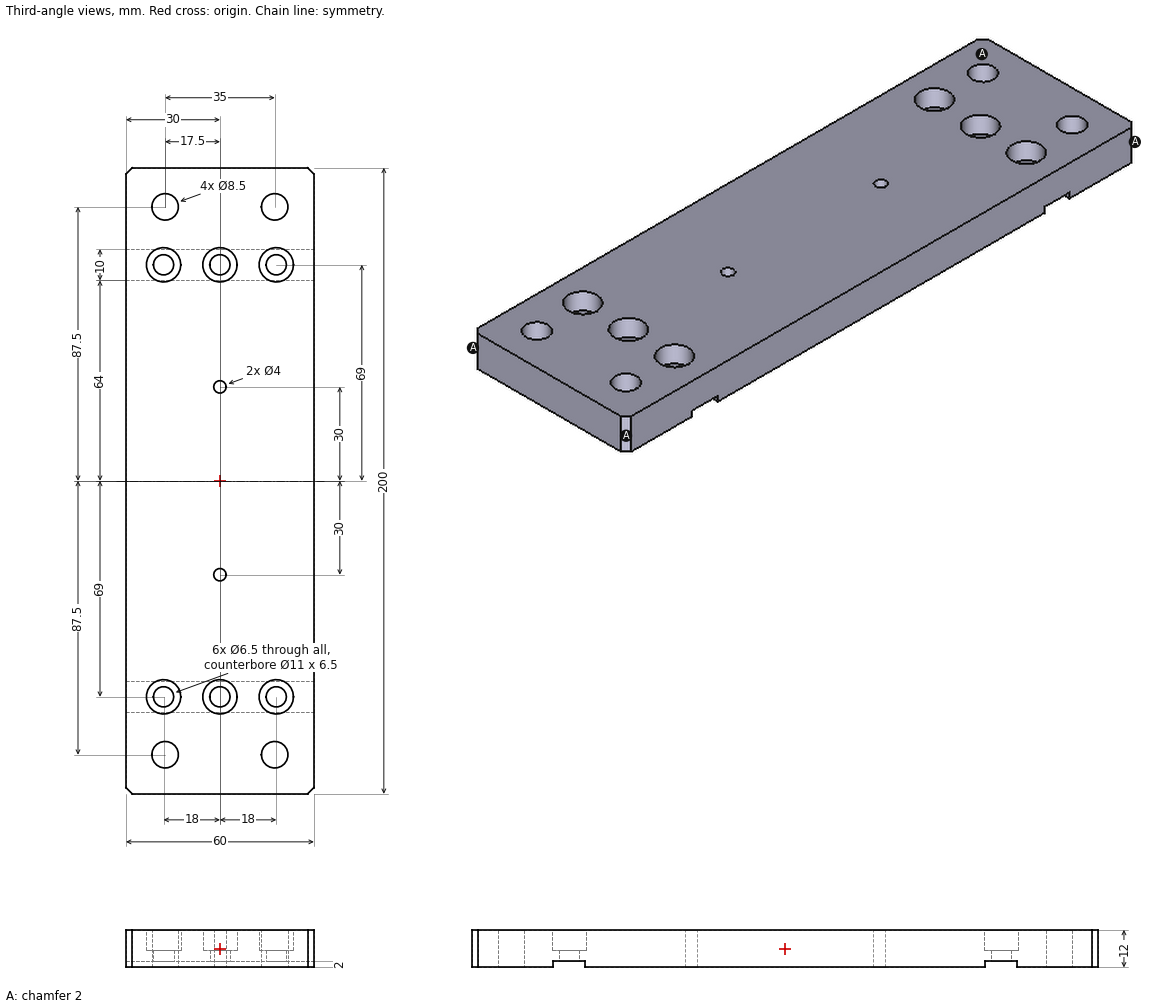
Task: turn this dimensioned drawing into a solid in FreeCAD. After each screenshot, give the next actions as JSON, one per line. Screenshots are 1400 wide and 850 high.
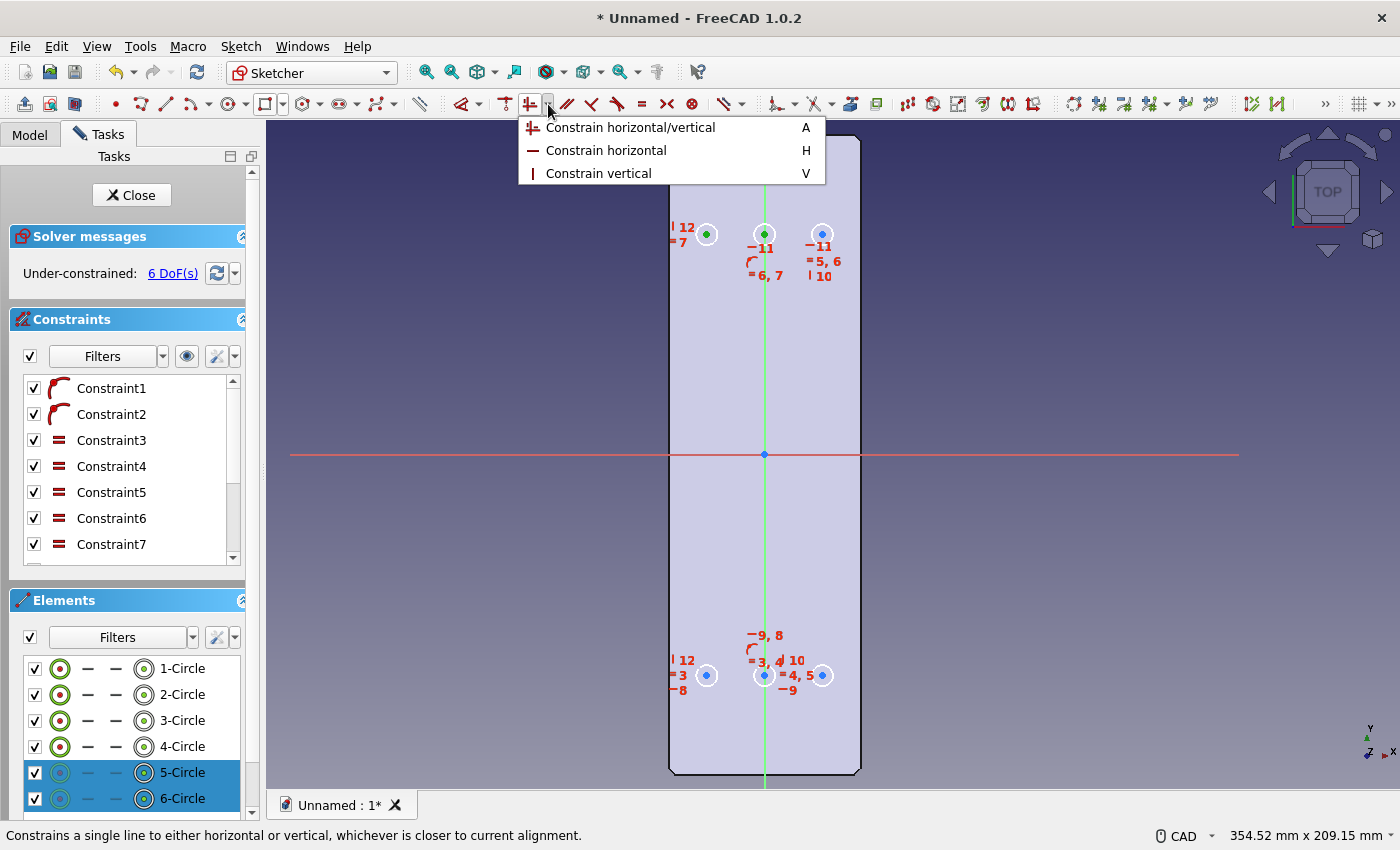
{"action": "left_click", "coordinate": [672, 150]}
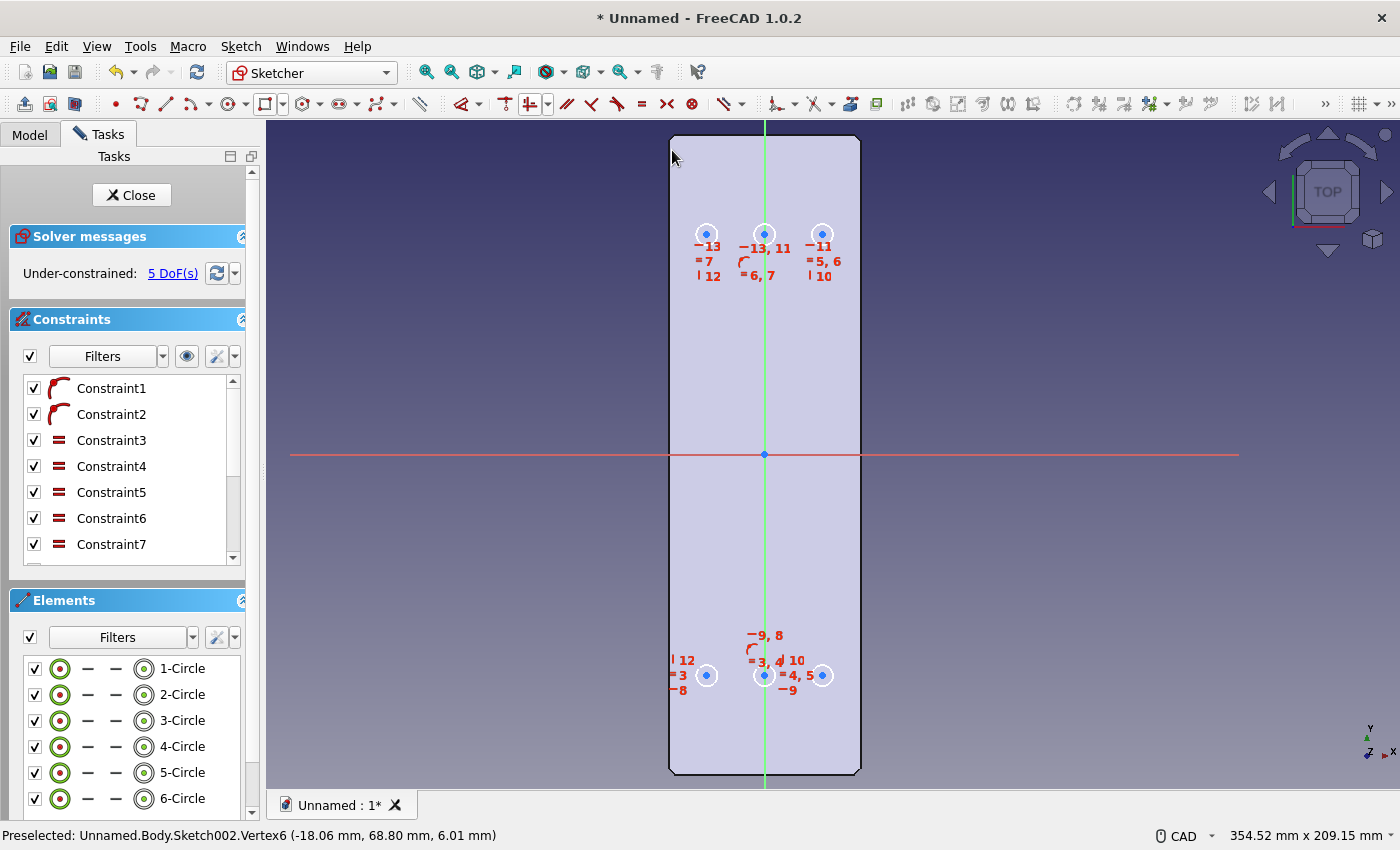
{"action": "left_click", "coordinate": [460, 104]}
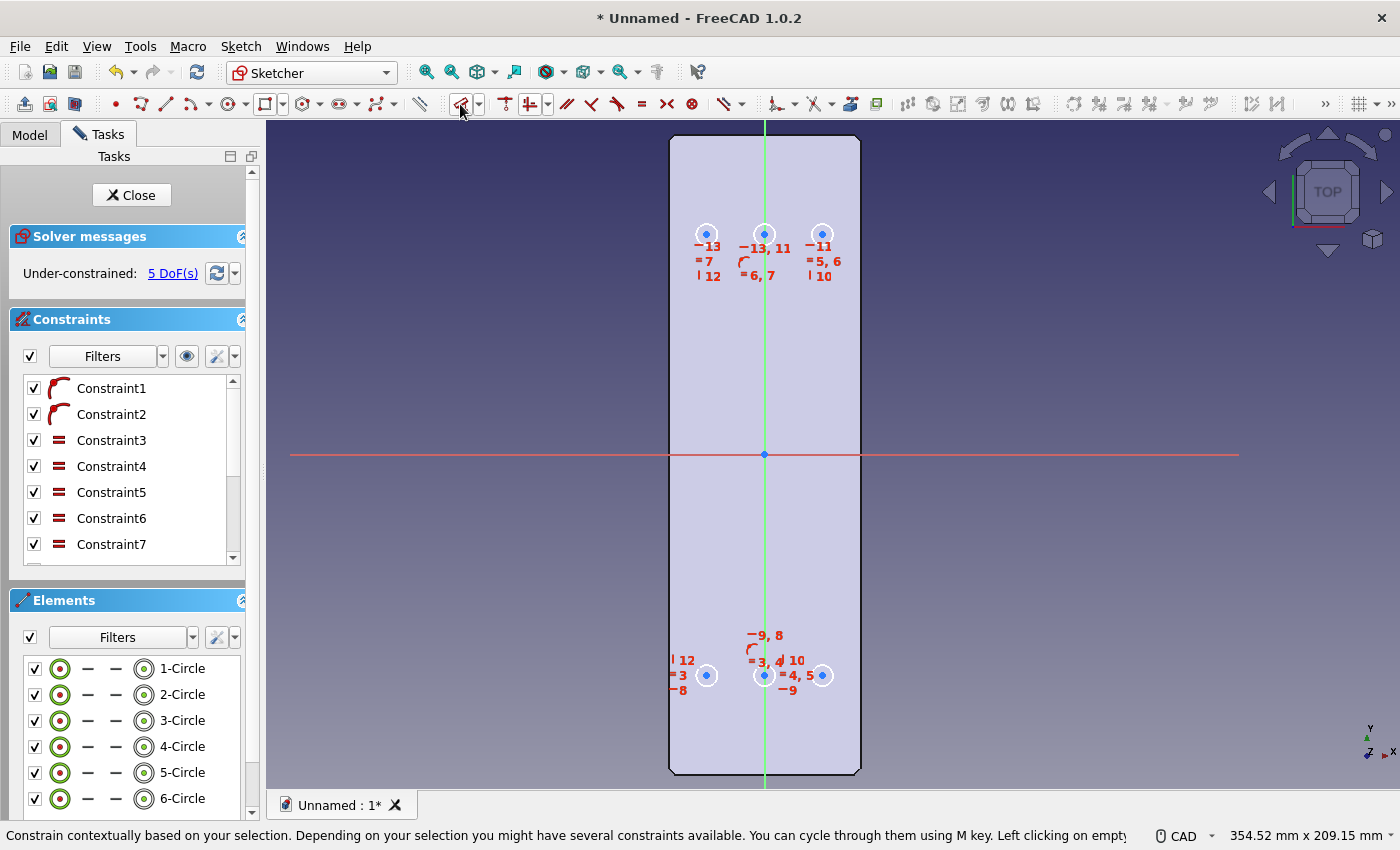
{"action": "scroll", "coordinate": [714, 668], "scroll_direction": "up", "scroll_amount": 4}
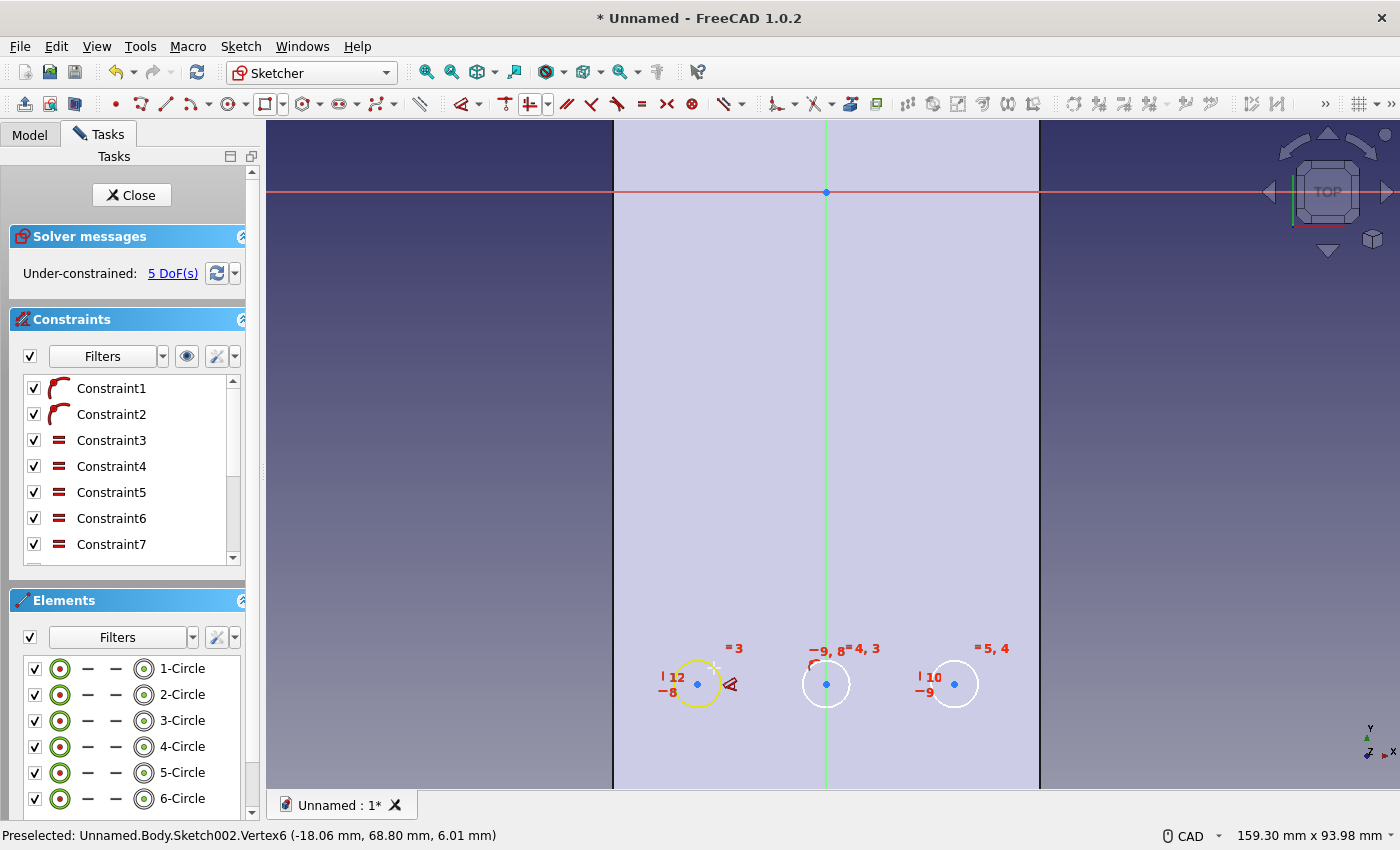
{"action": "left_click", "coordinate": [714, 668]}
{"action": "left_click", "coordinate": [737, 646]}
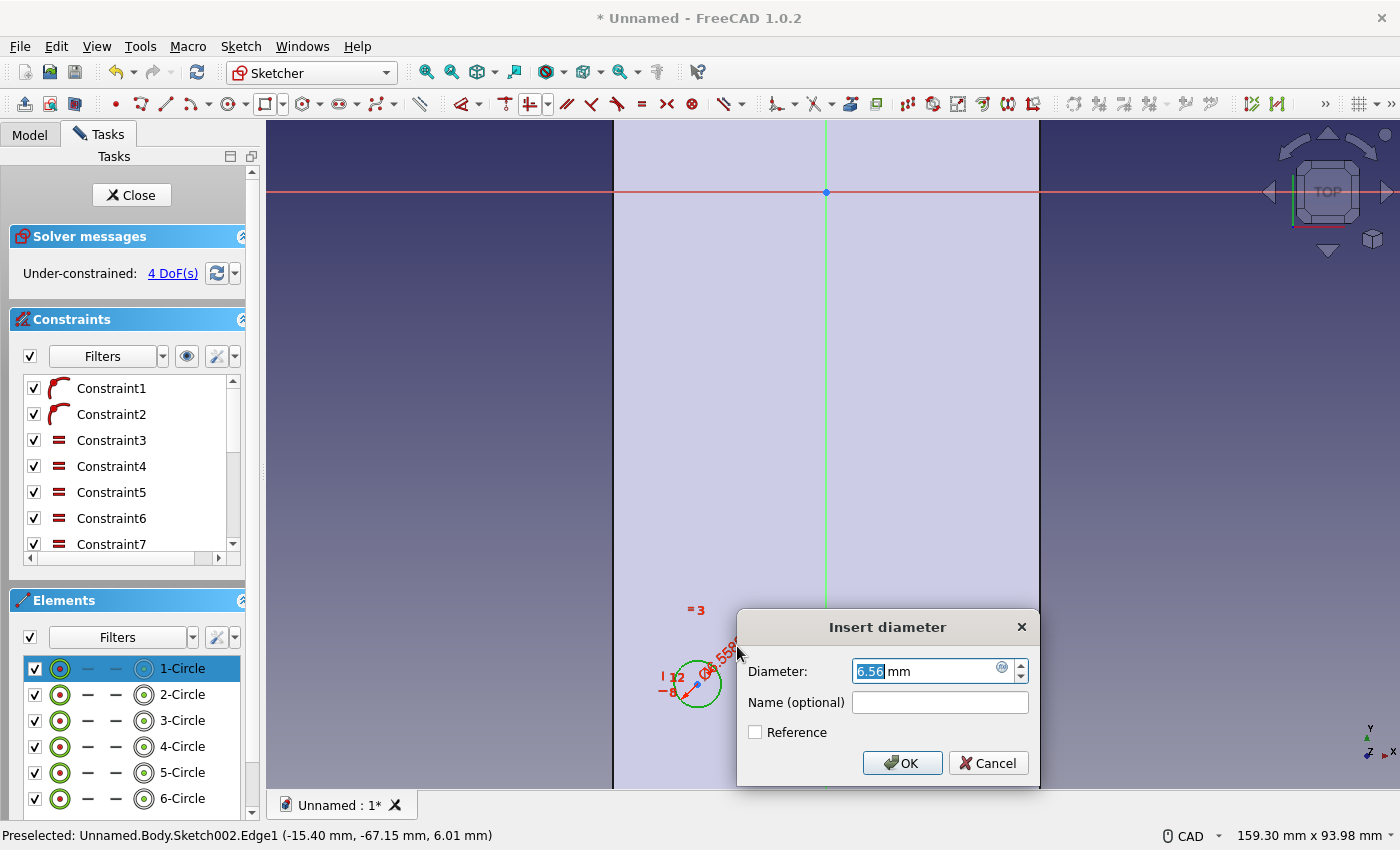
{"action": "type", "text": "6.5"}
{"action": "key", "text": "Return"}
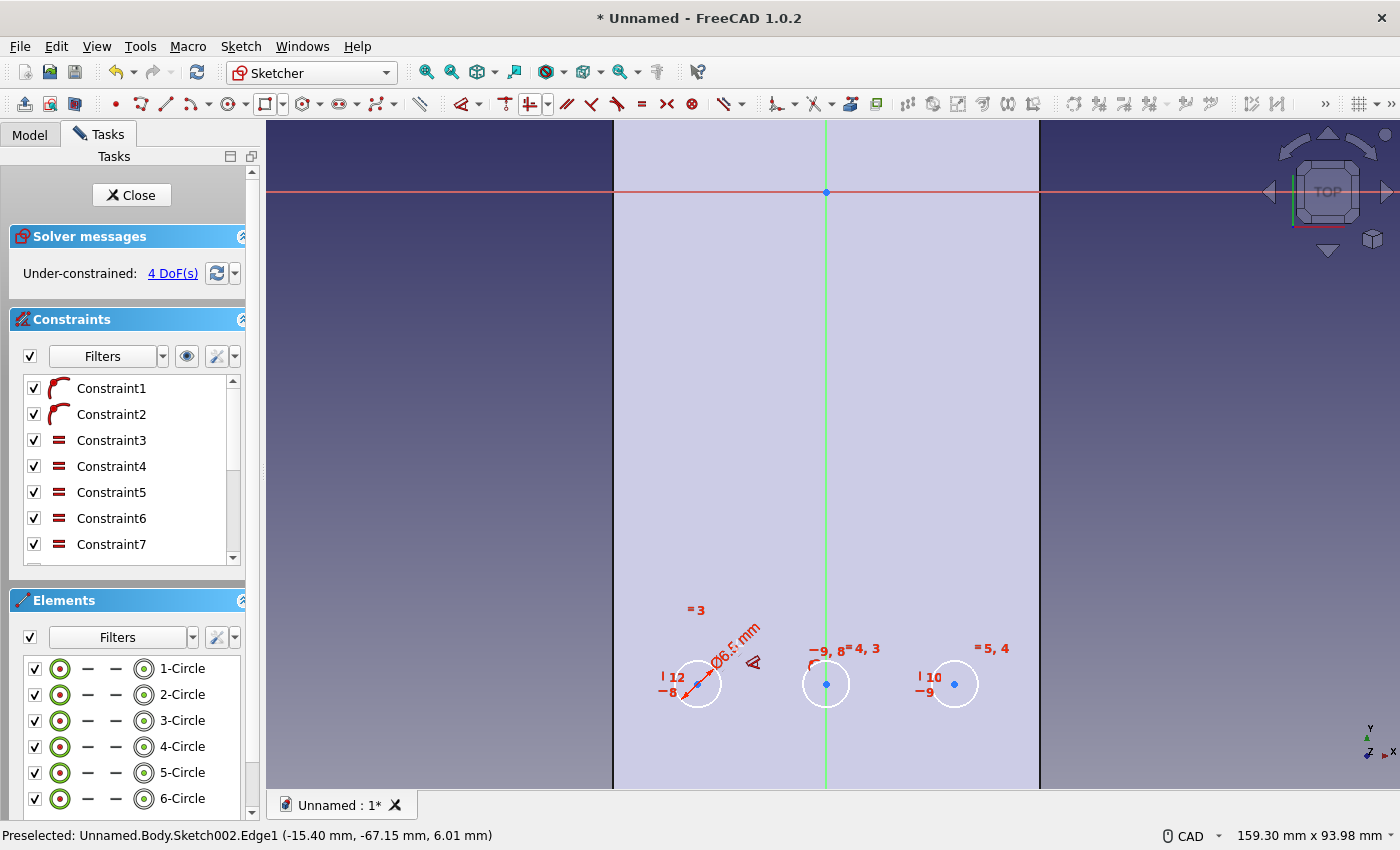
{"action": "left_click", "coordinate": [698, 684]}
{"action": "left_click", "coordinate": [762, 718]}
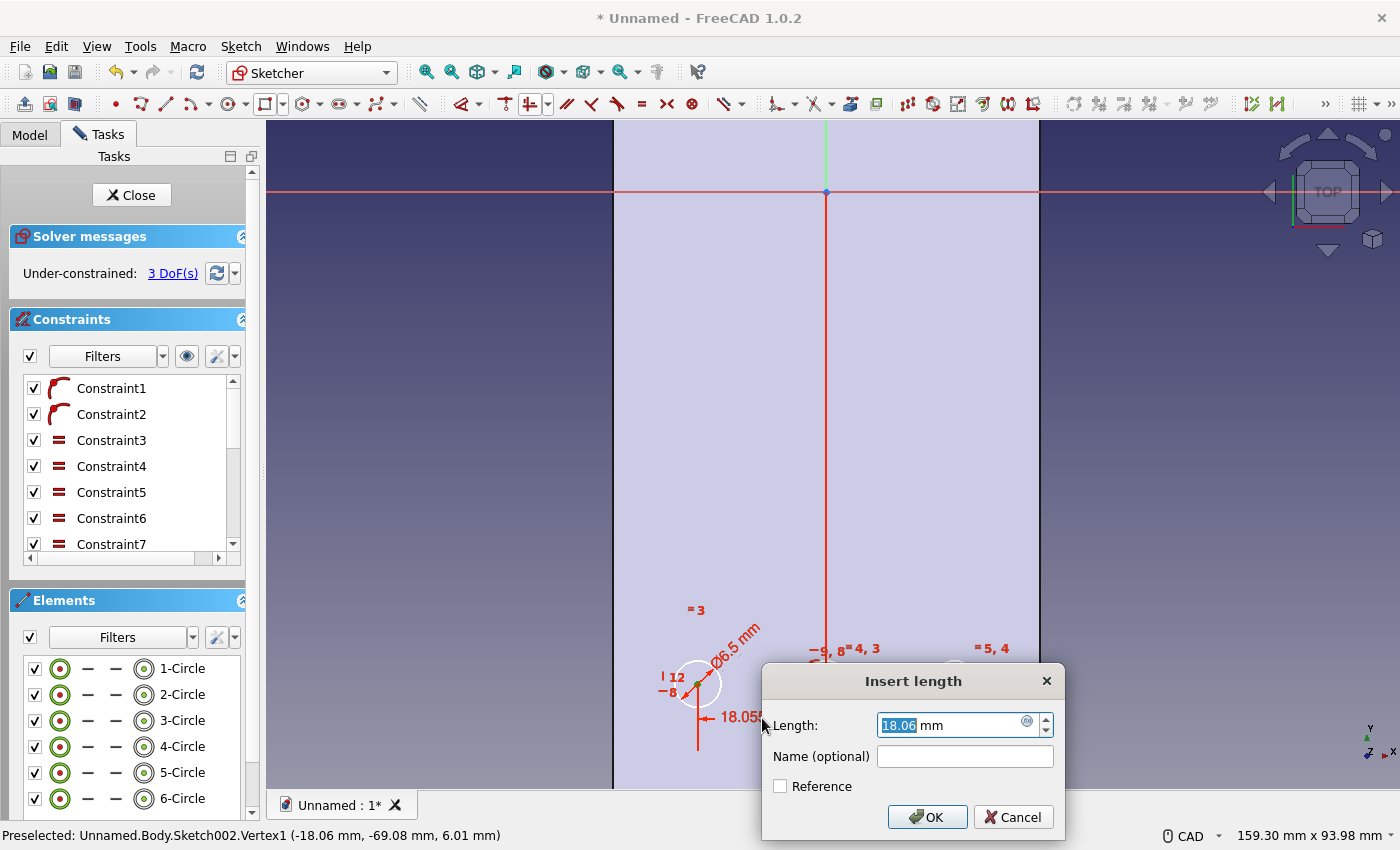
{"action": "type", "text": "18"}
{"action": "key", "text": "Return"}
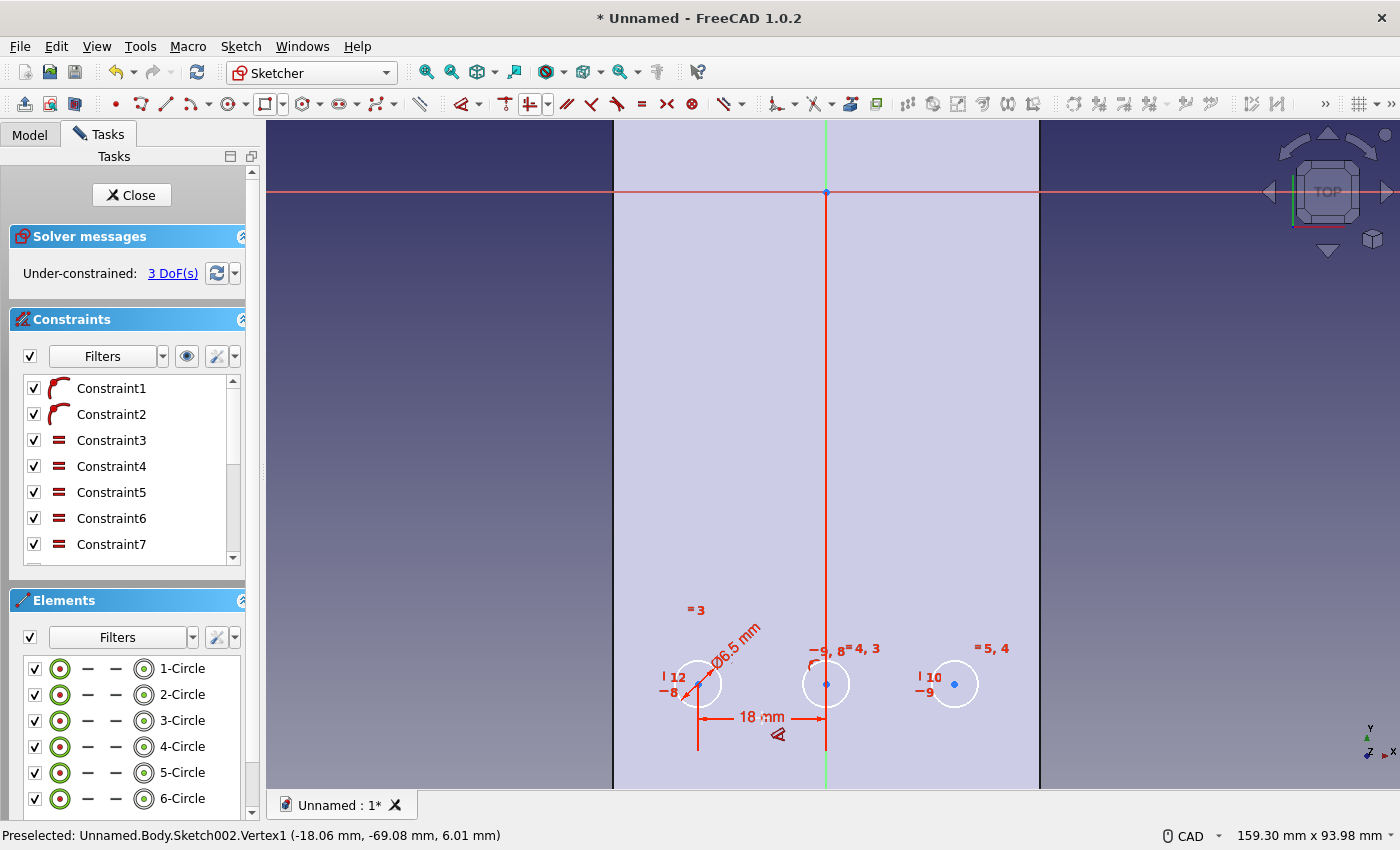
{"action": "left_click", "coordinate": [698, 684]}
{"action": "left_click", "coordinate": [664, 438]}